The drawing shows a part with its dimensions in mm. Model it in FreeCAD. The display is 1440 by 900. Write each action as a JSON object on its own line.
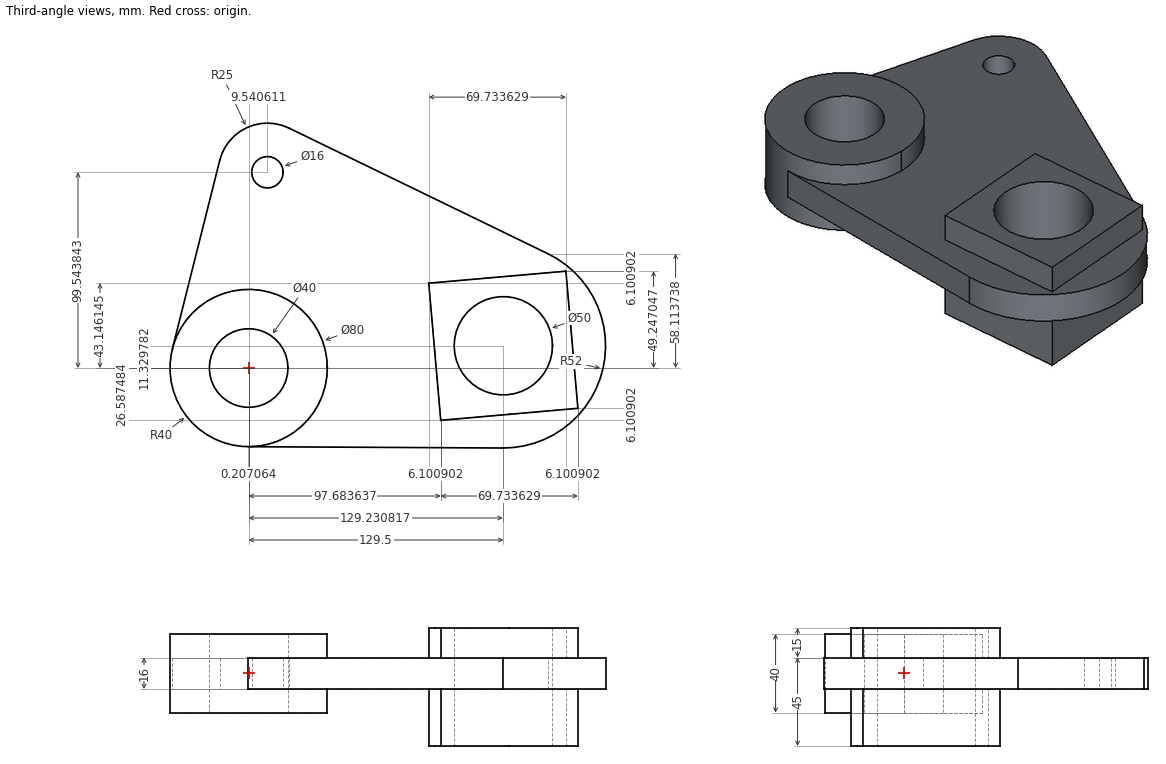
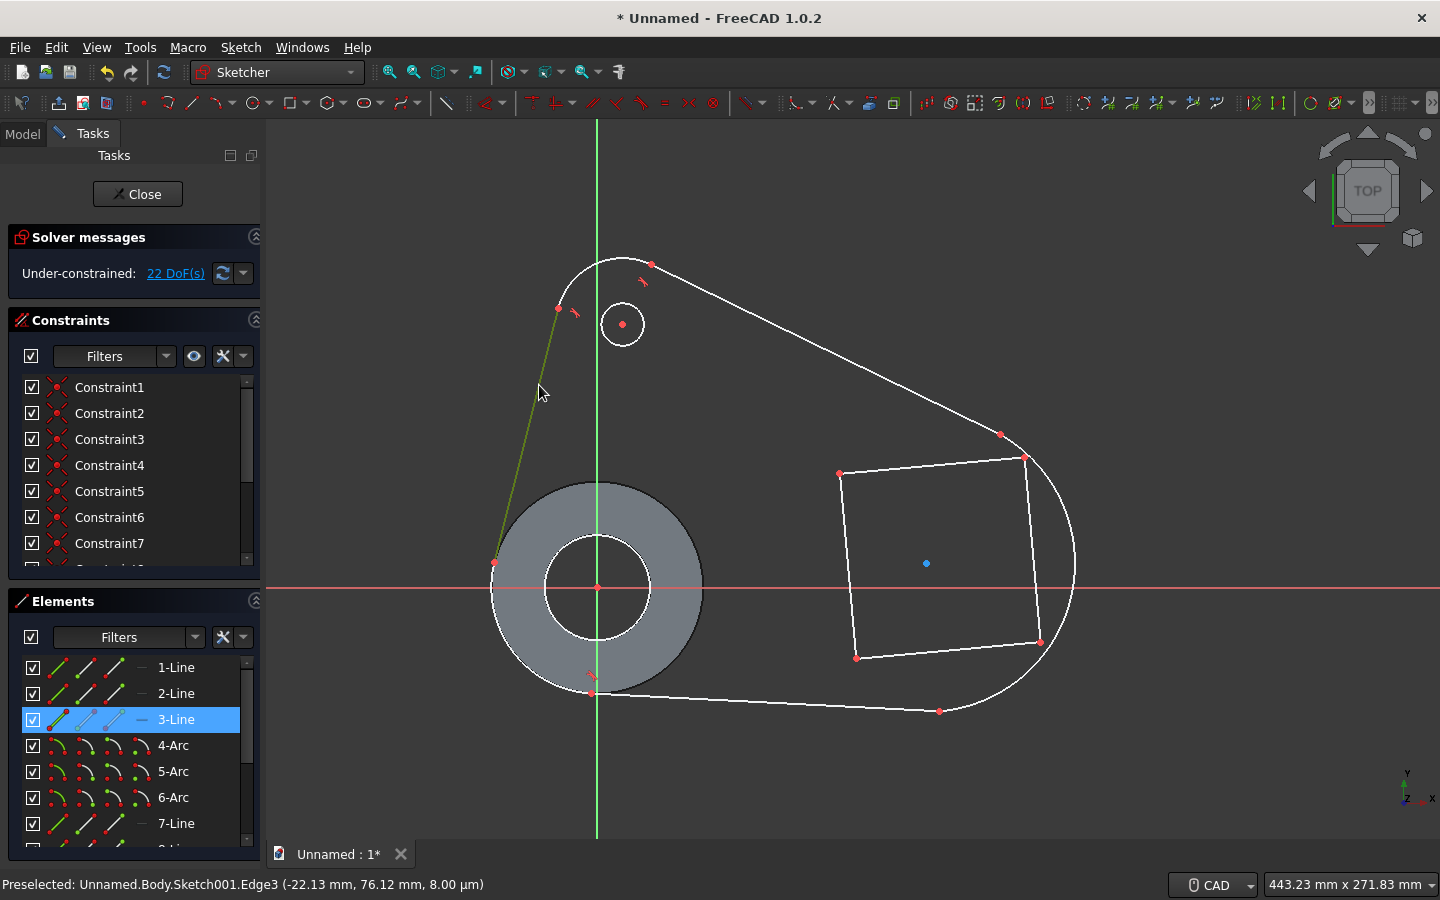
{"action": "left_click", "coordinate": [496, 618]}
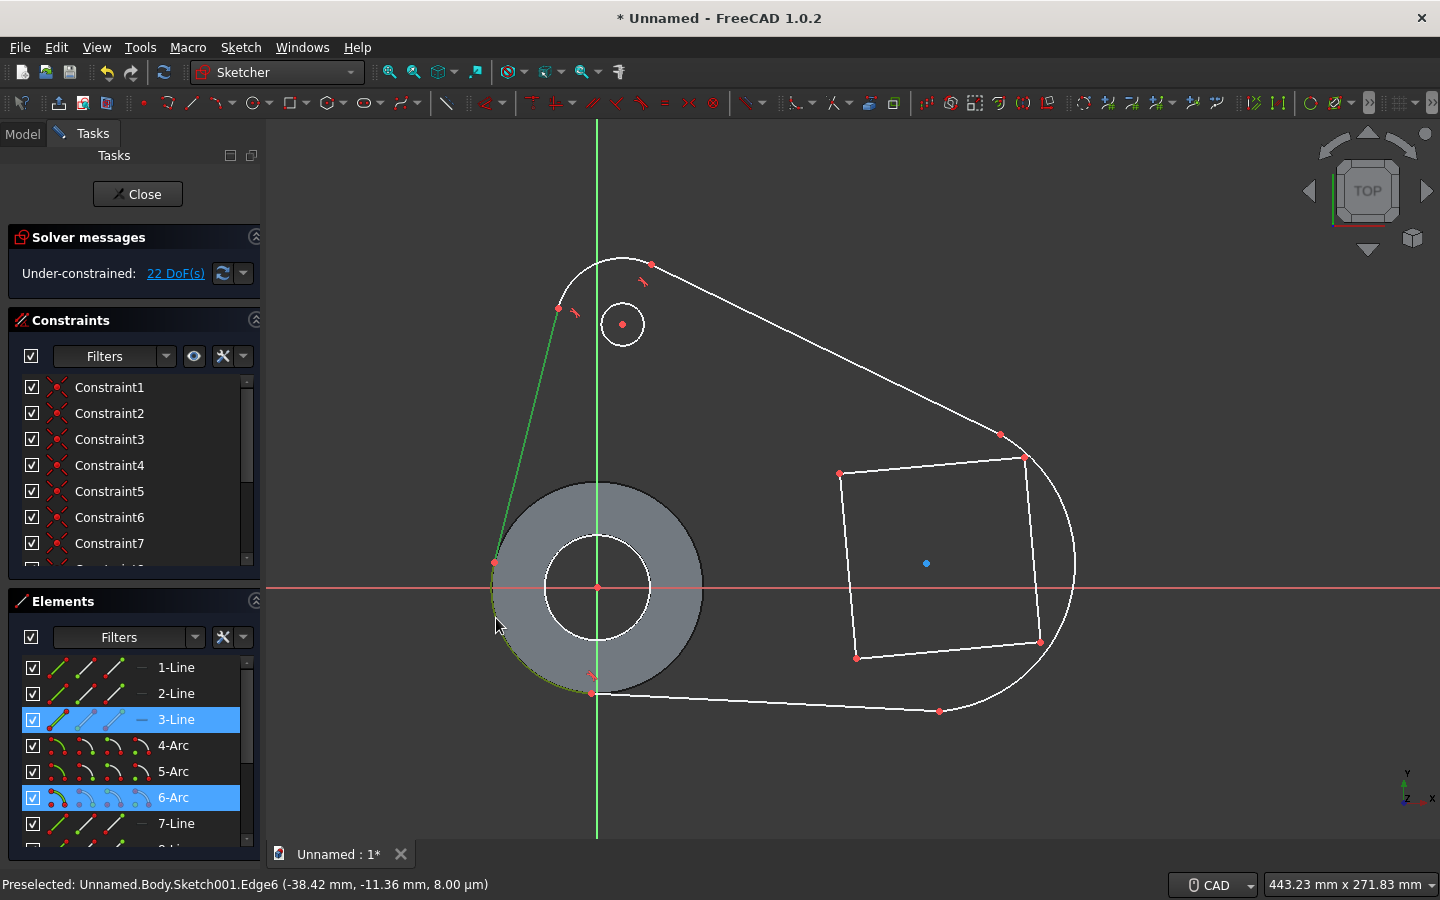
{"action": "key", "text": "t"}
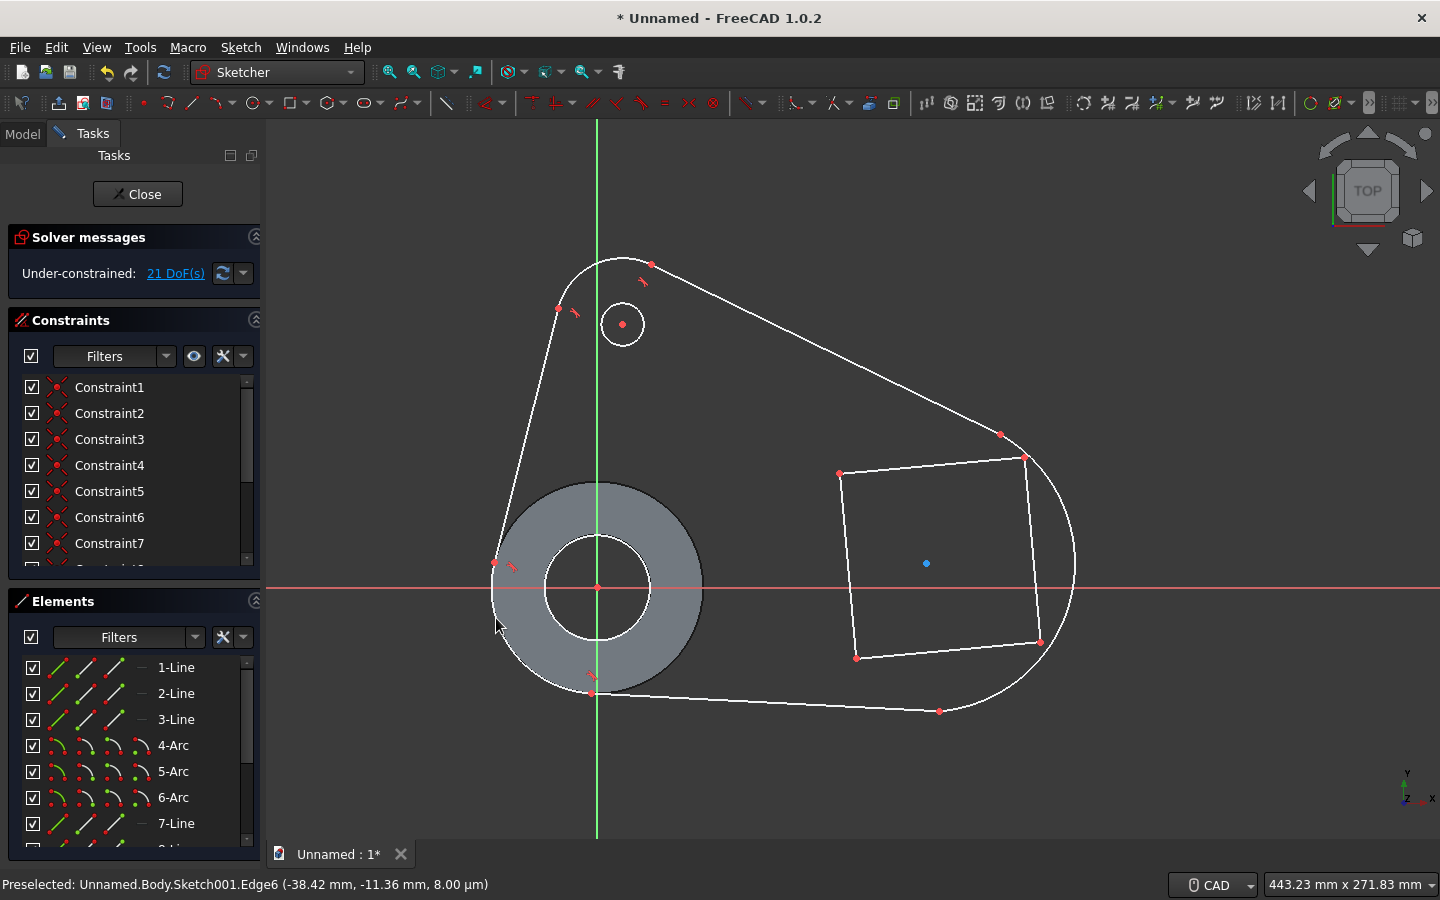
{"action": "scroll", "coordinate": [597, 588], "scroll_direction": "up", "scroll_amount": 4}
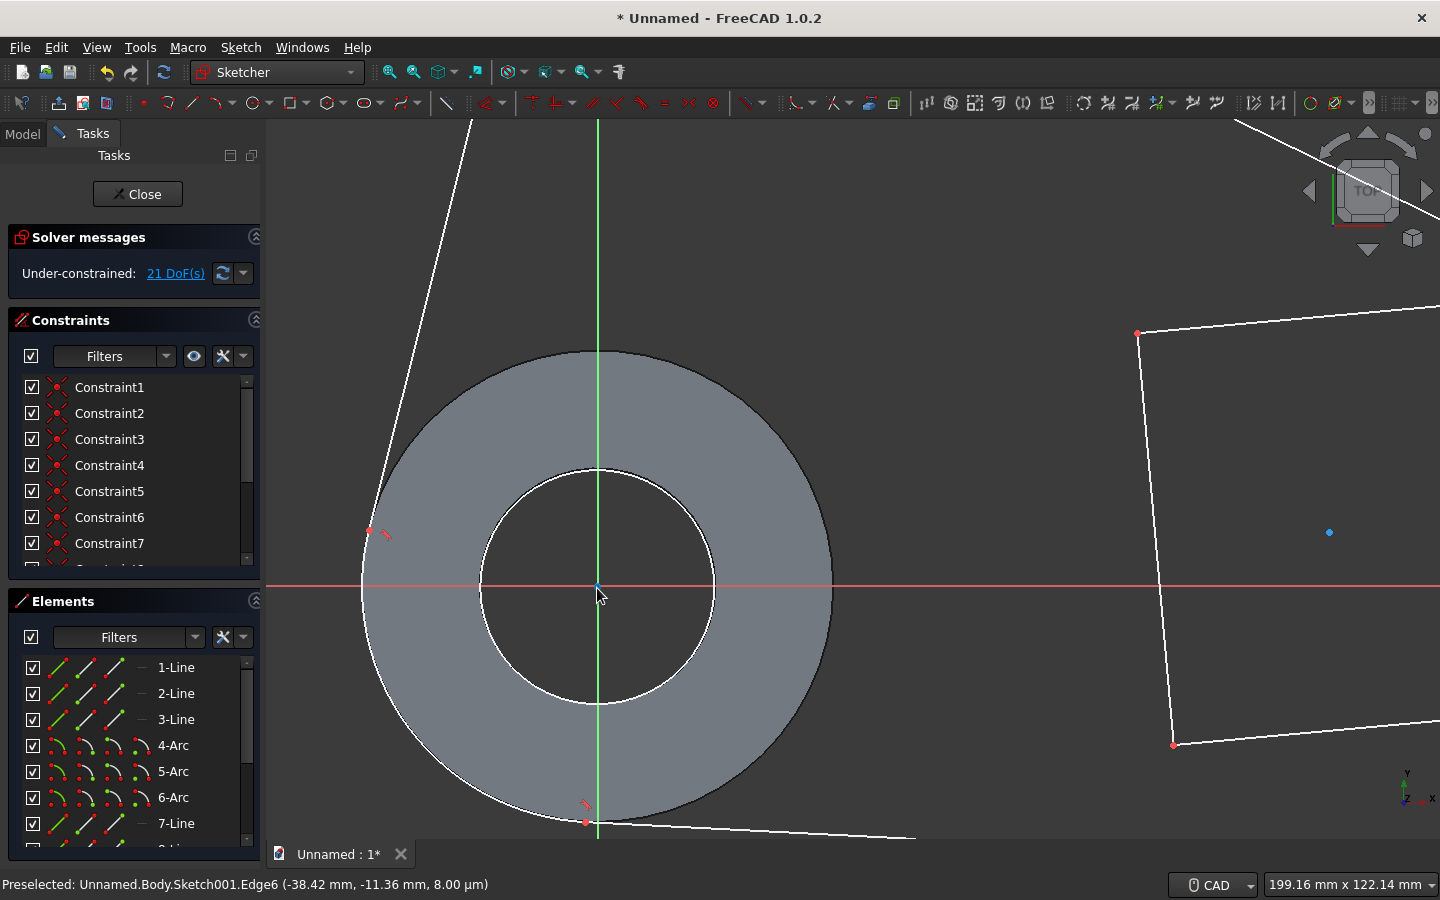
{"action": "left_click_drag", "start_coordinate": [587, 576], "coordinate": [608, 597]}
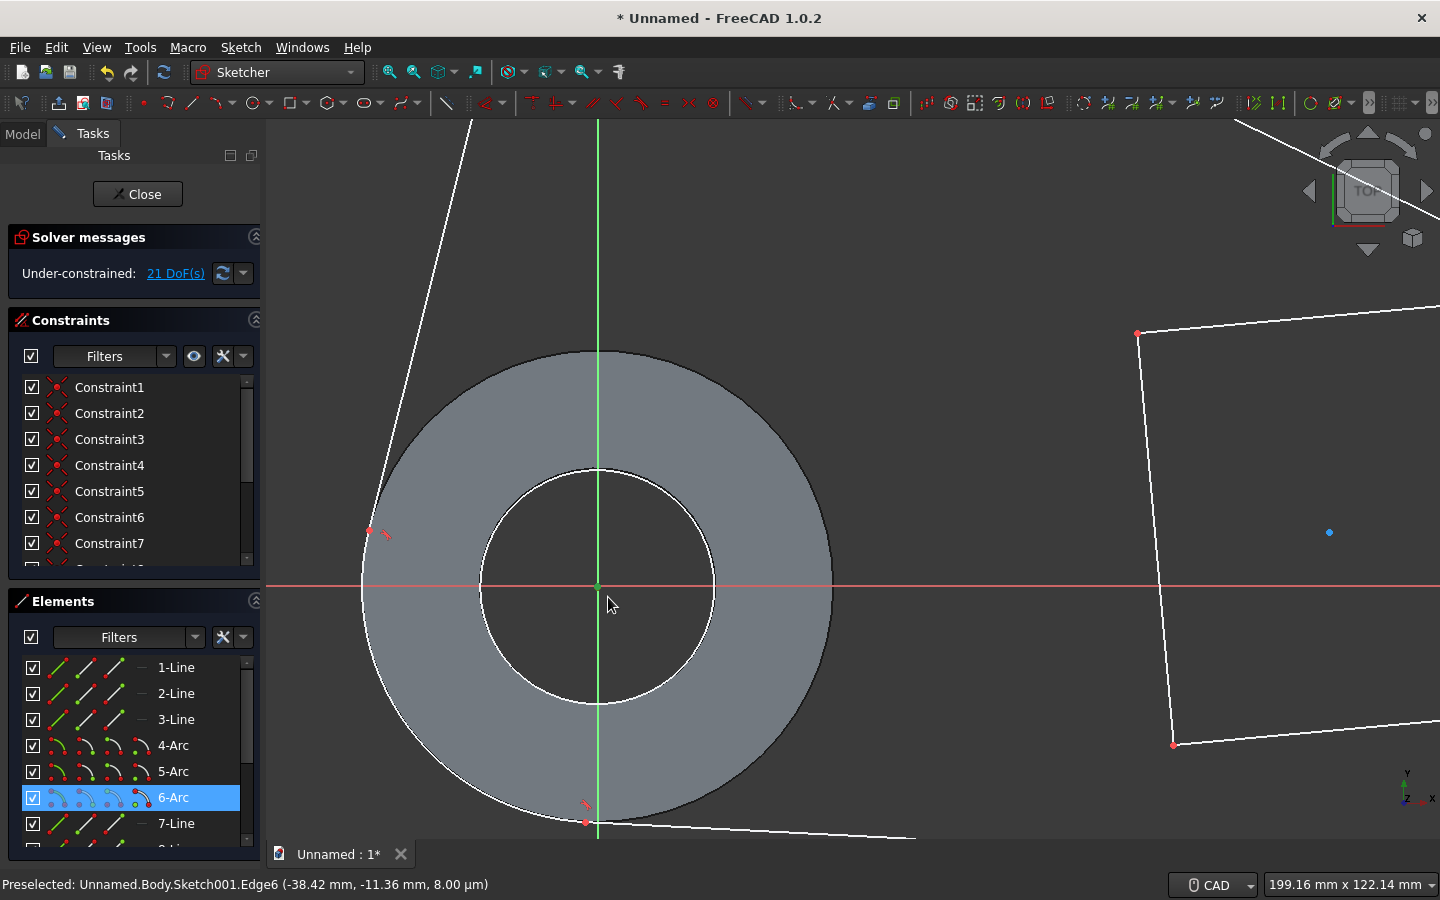
{"action": "key", "text": "c"}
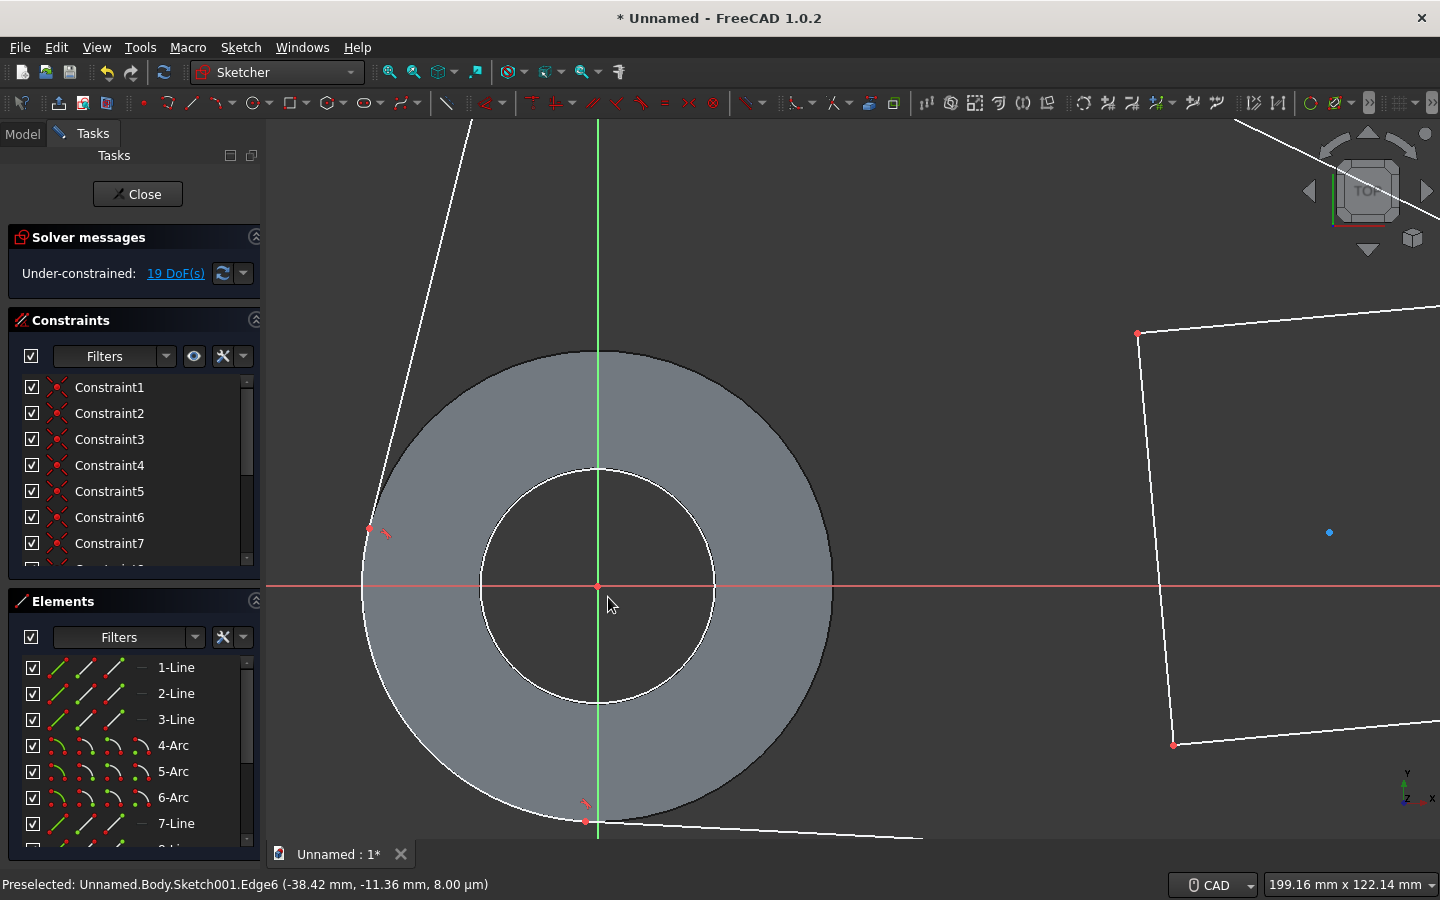
{"action": "left_click", "coordinate": [486, 104]}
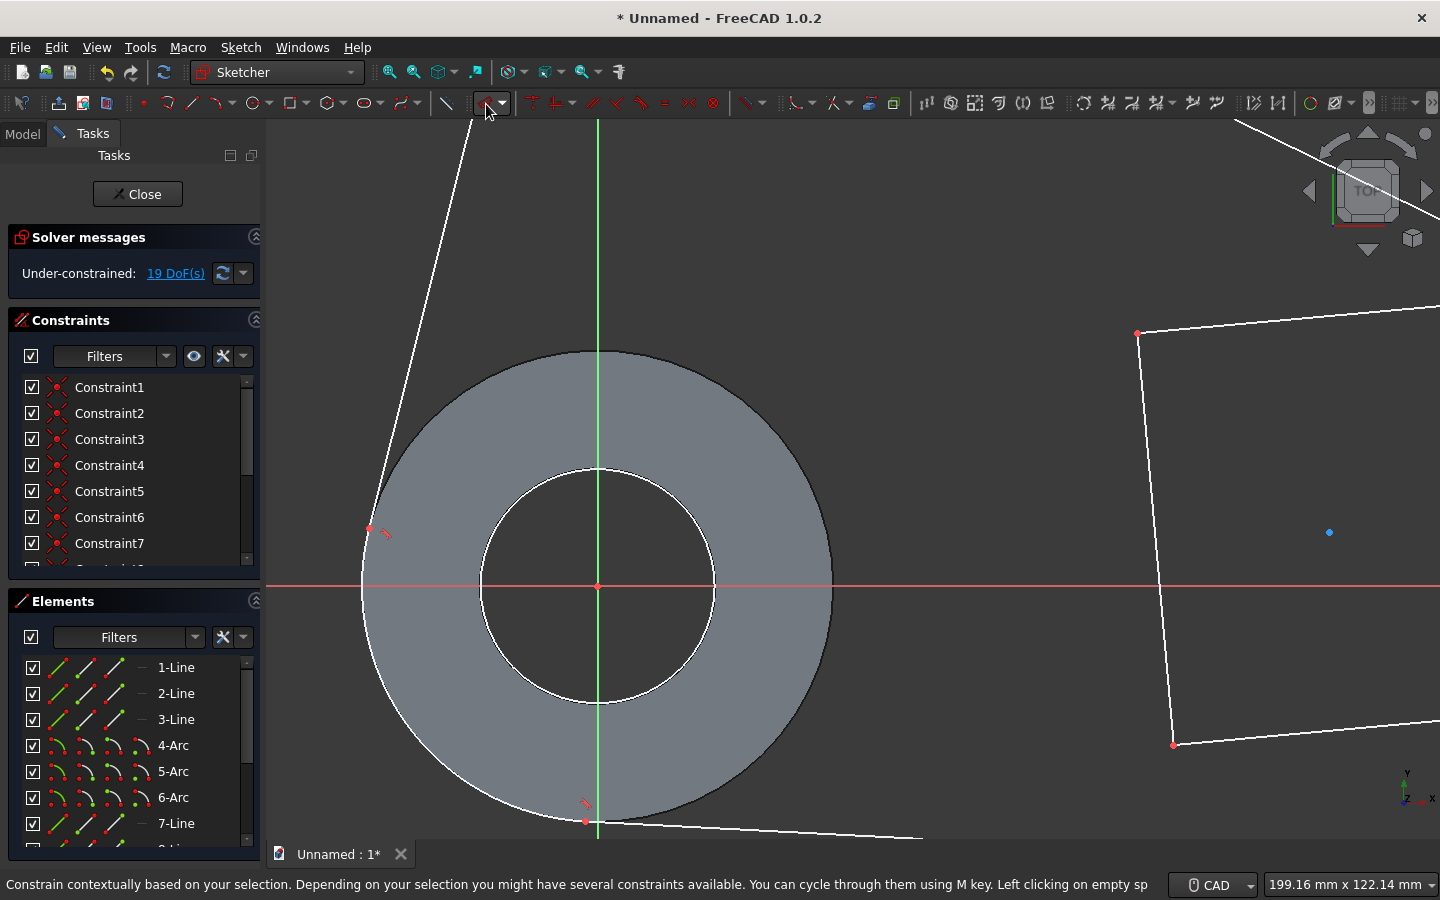
{"action": "scroll", "coordinate": [597, 588], "scroll_direction": "down", "scroll_amount": 4}